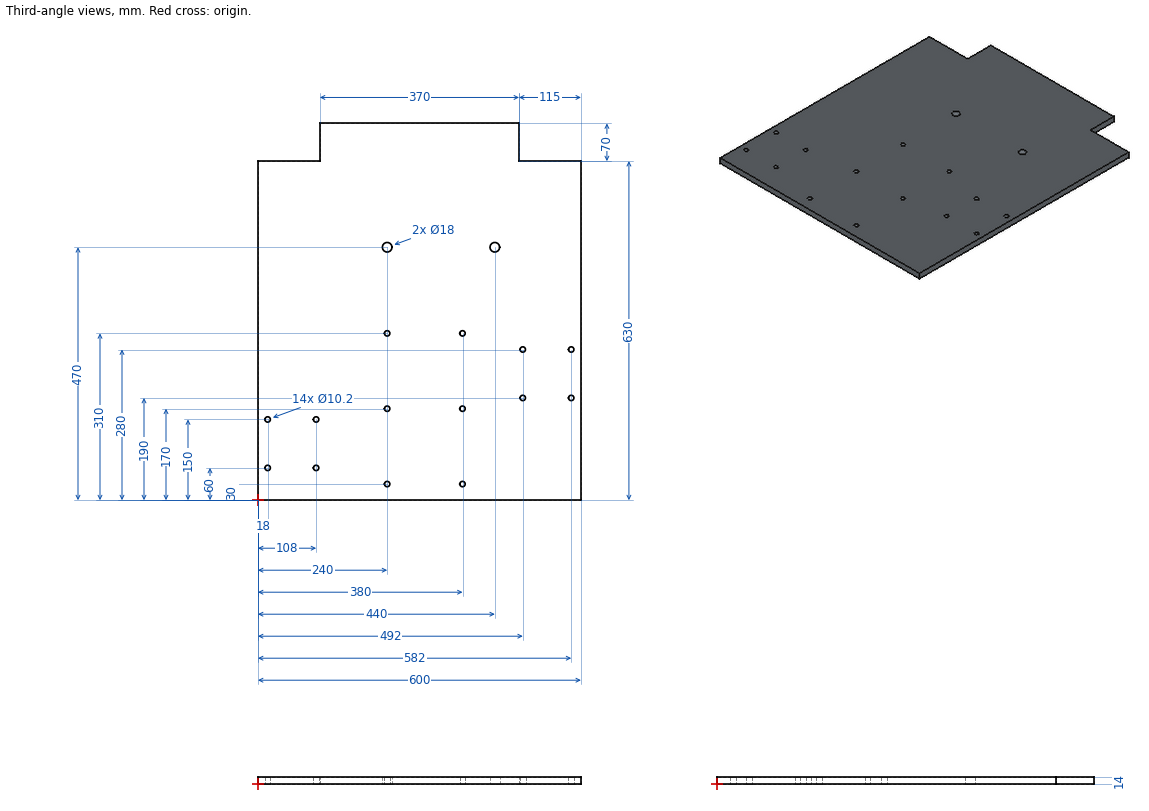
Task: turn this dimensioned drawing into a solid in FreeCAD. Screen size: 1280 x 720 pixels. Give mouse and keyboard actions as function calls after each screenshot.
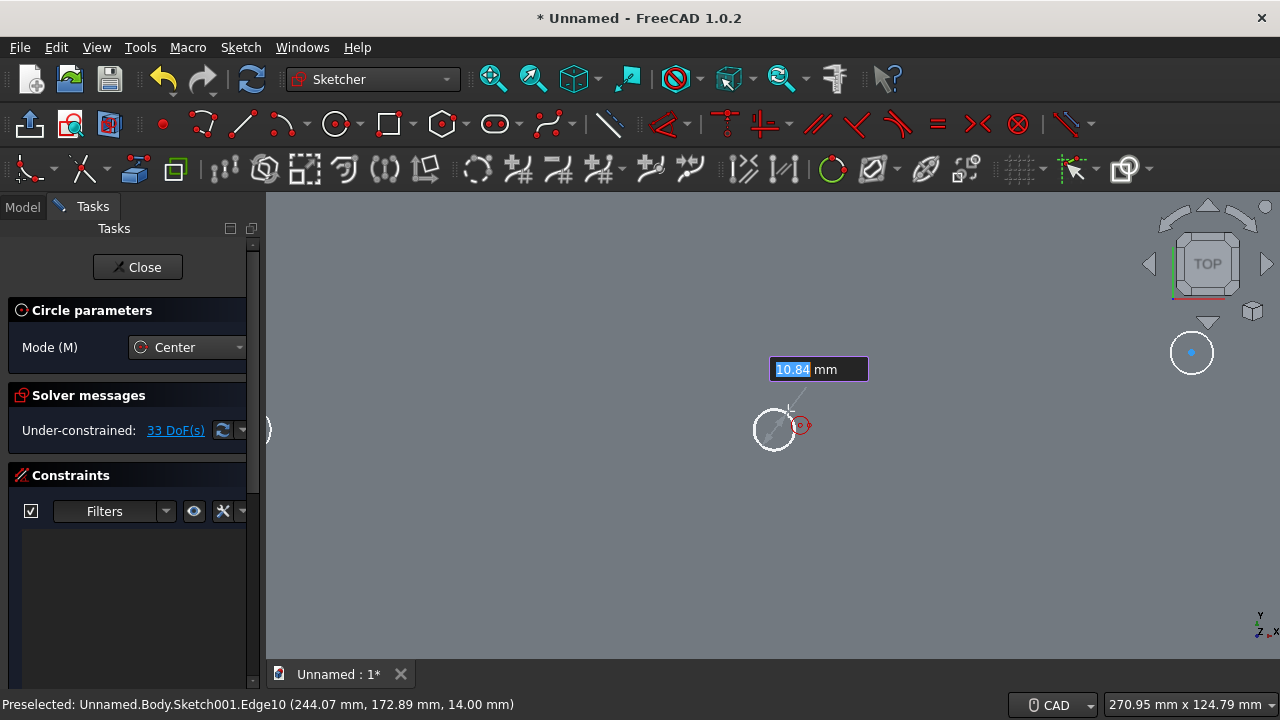
click(786, 411)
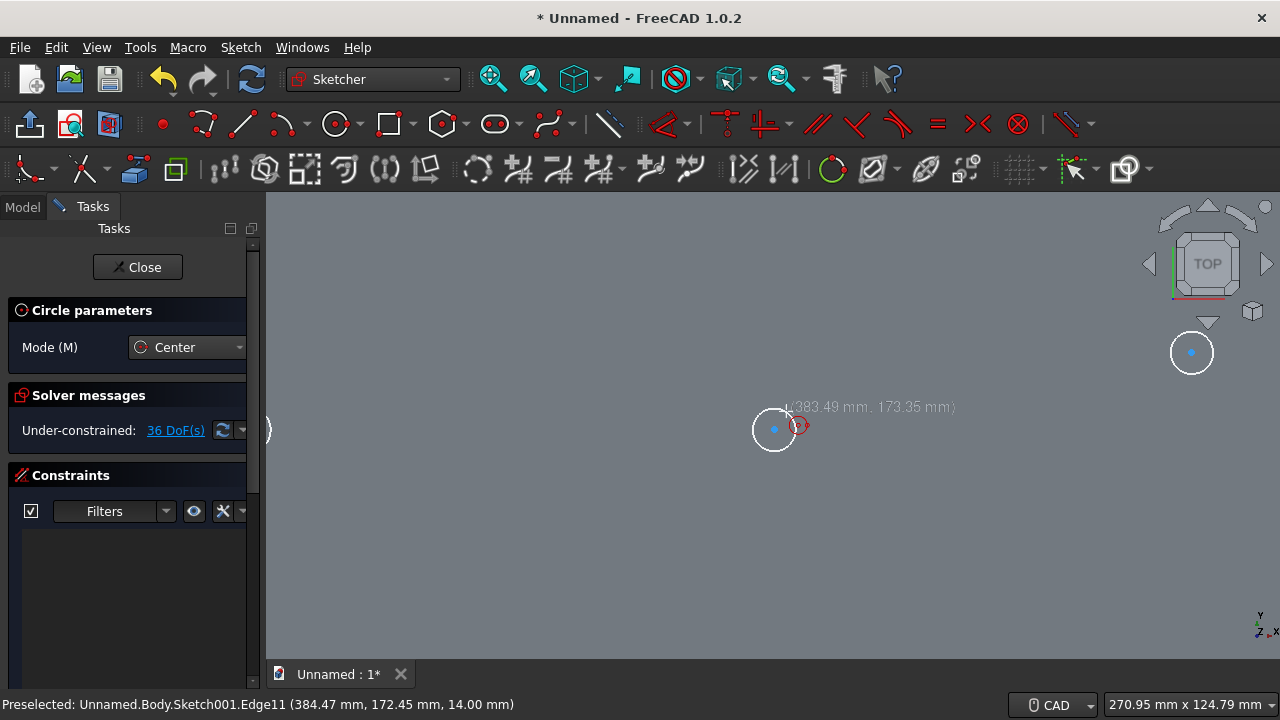
scroll(788, 411, down, 7)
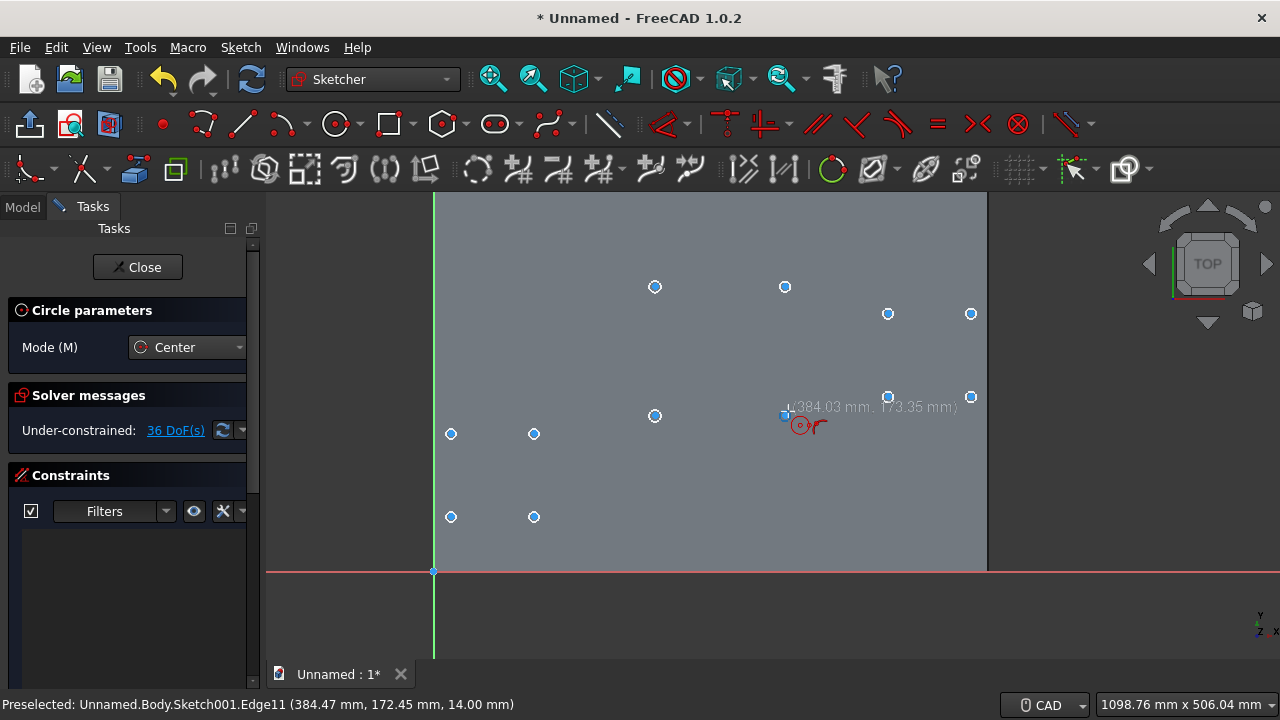
scroll(655, 544, up, 8)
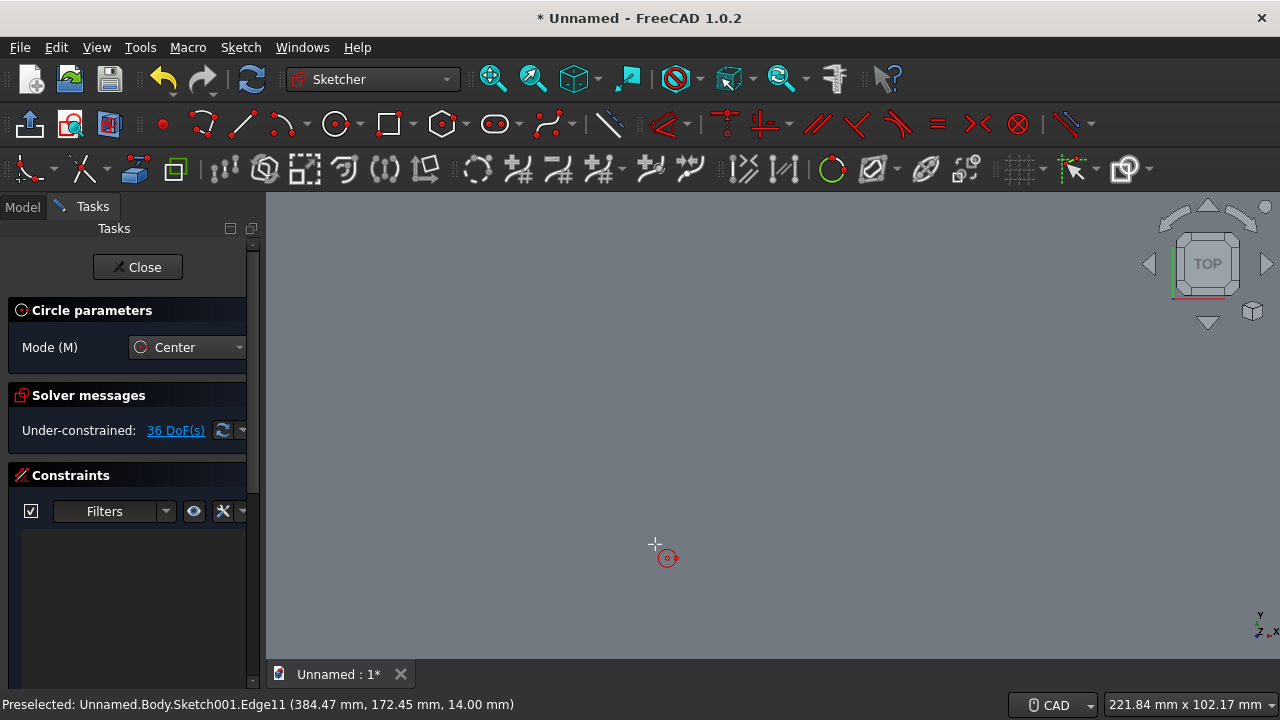
scroll(655, 544, down, 8)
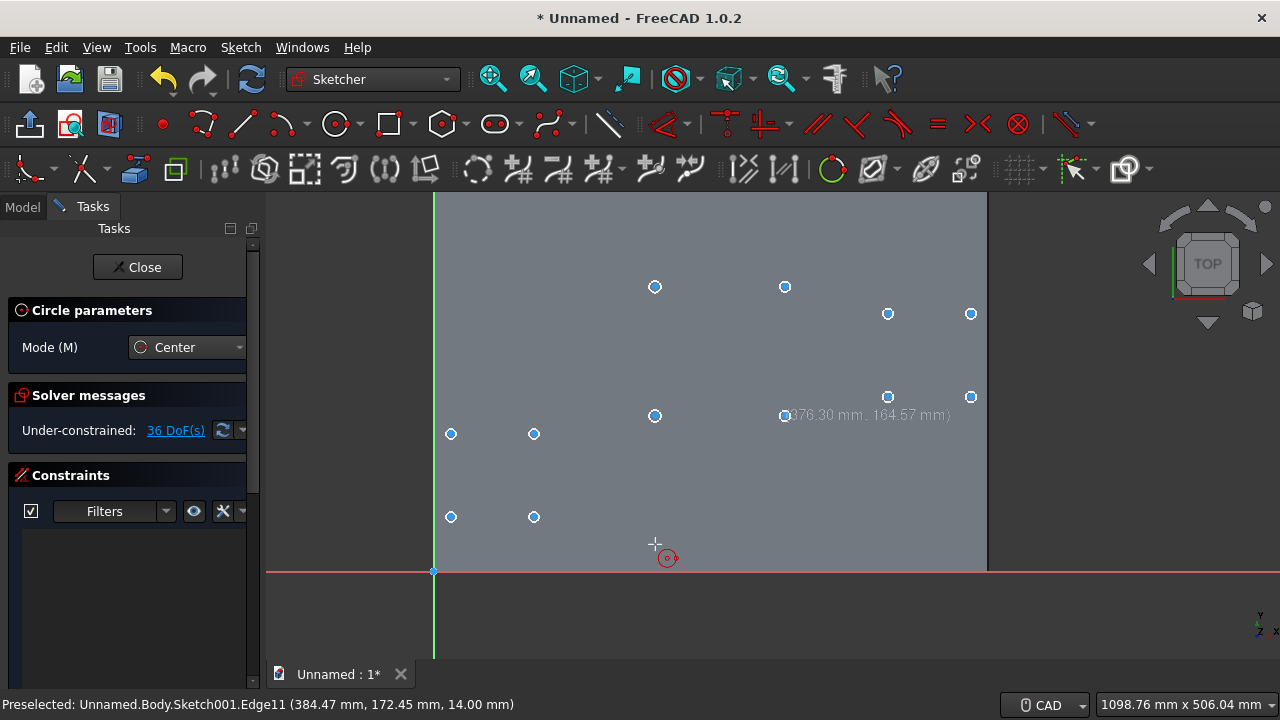
click(655, 544)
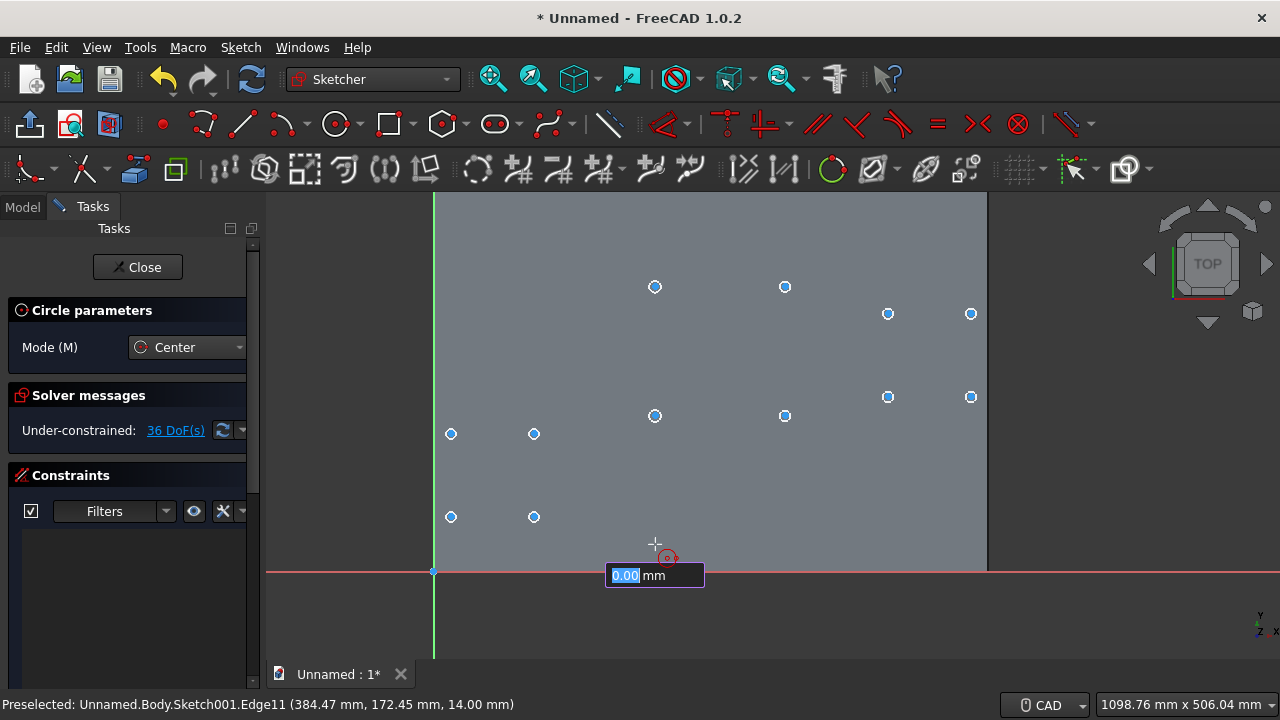
scroll(659, 541, up, 7)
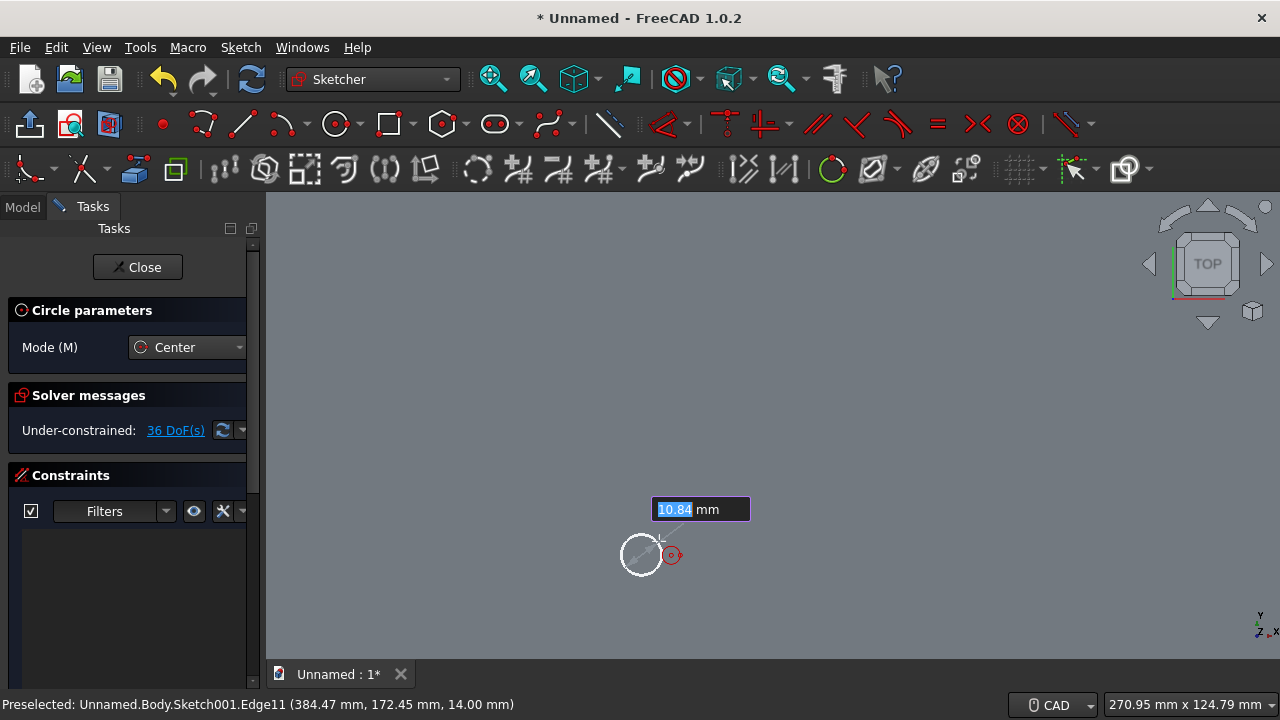
click(657, 537)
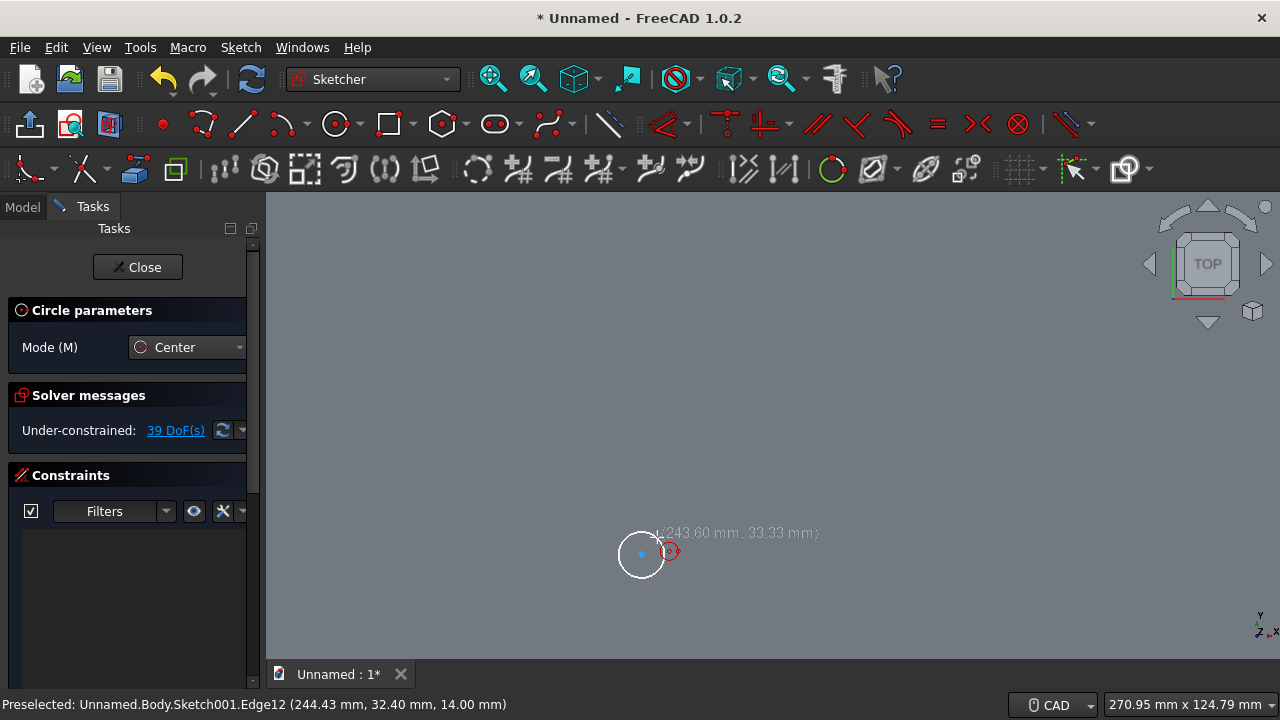
scroll(659, 541, down, 7)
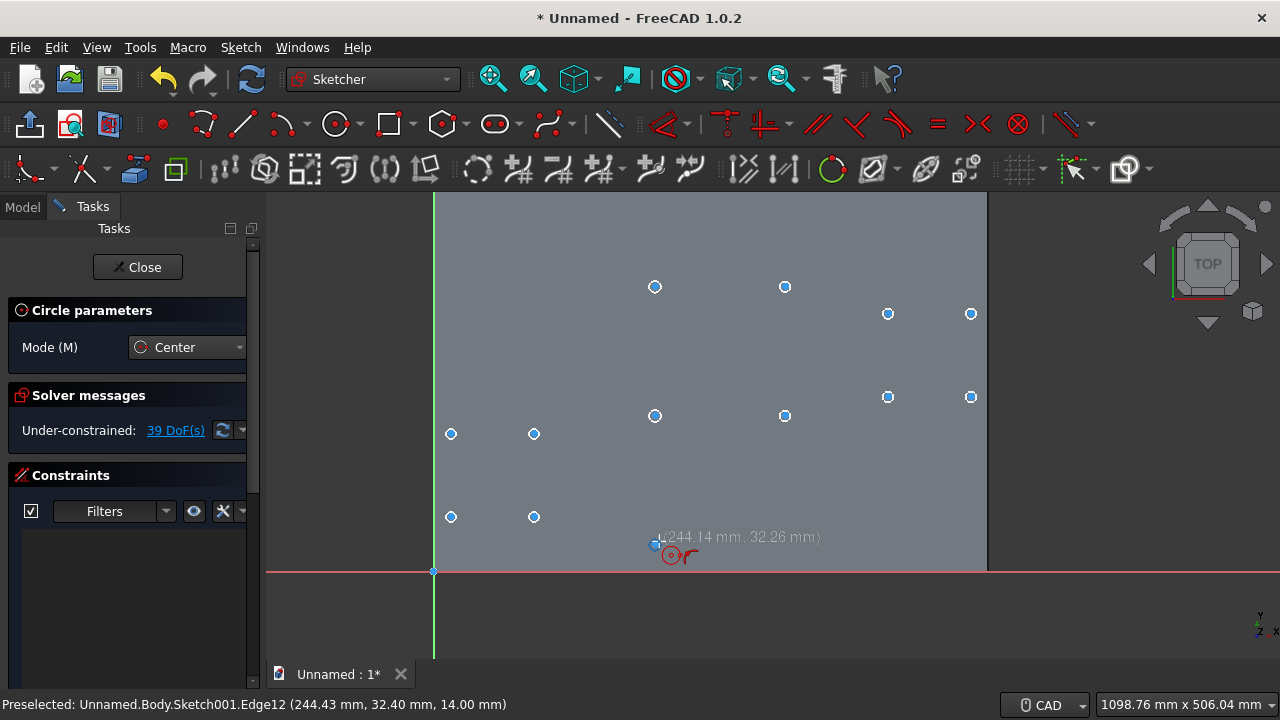
scroll(785, 544, up, 8)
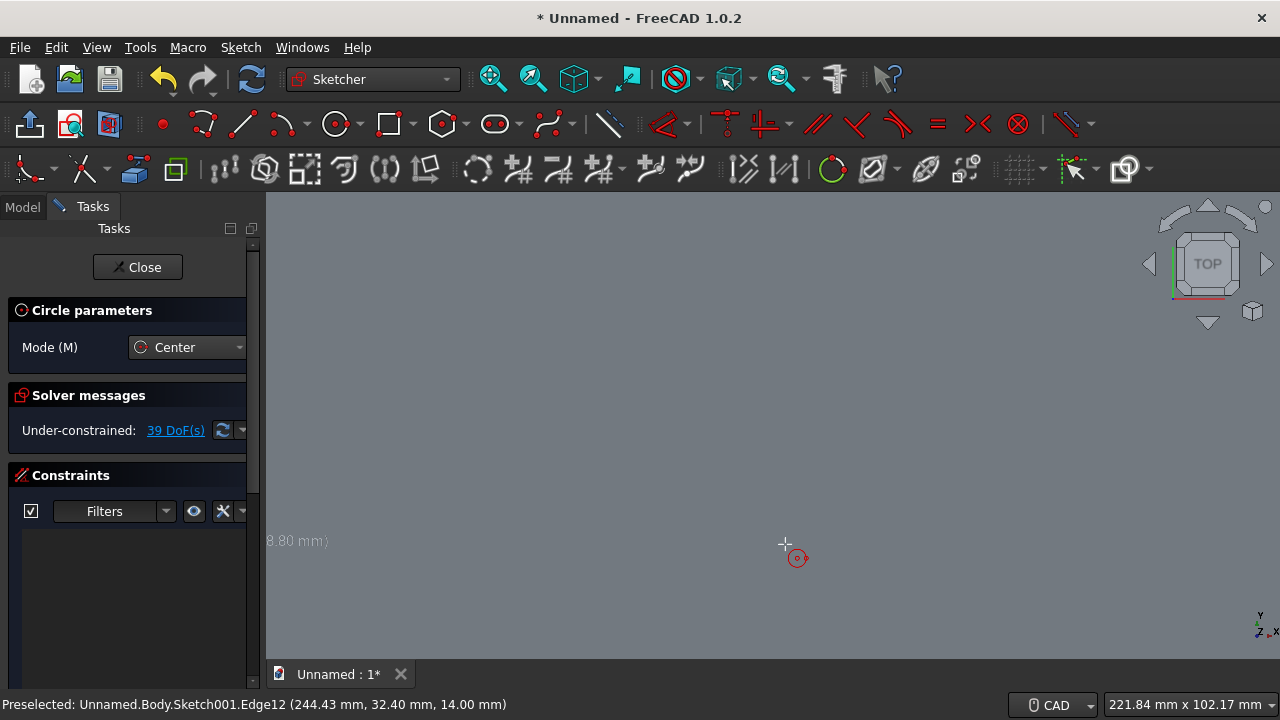
scroll(785, 544, down, 8)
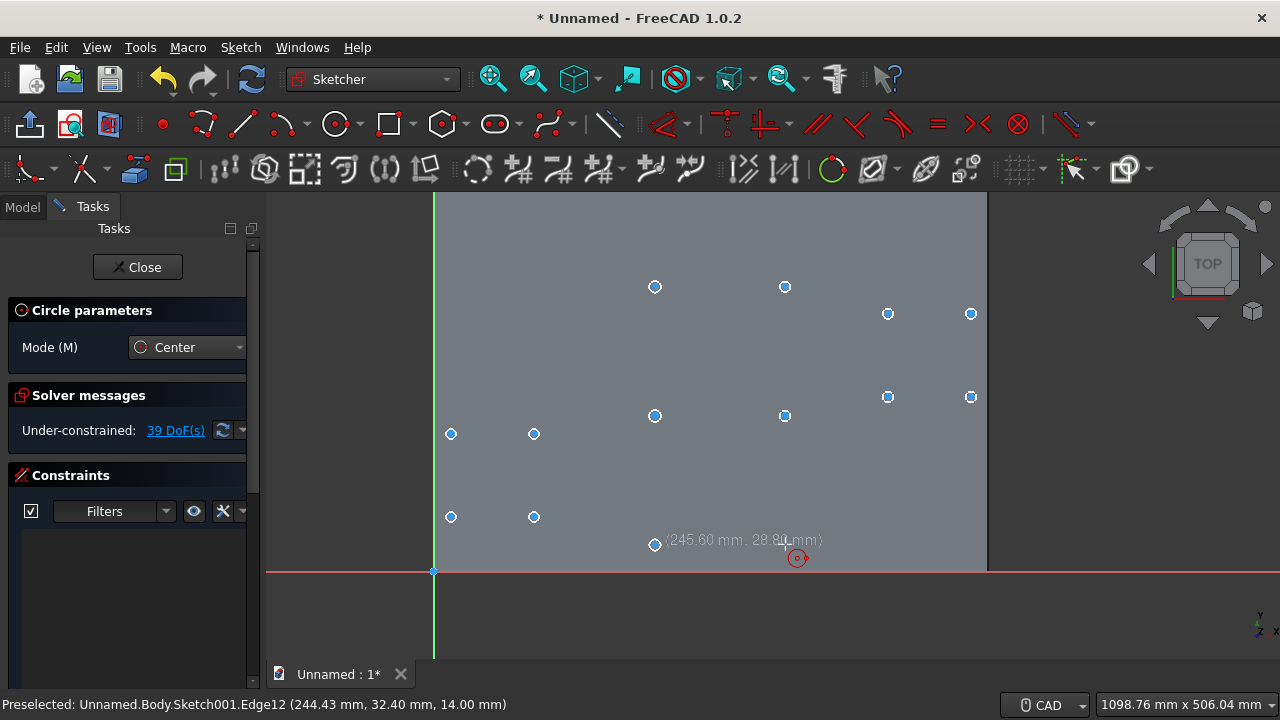
click(785, 544)